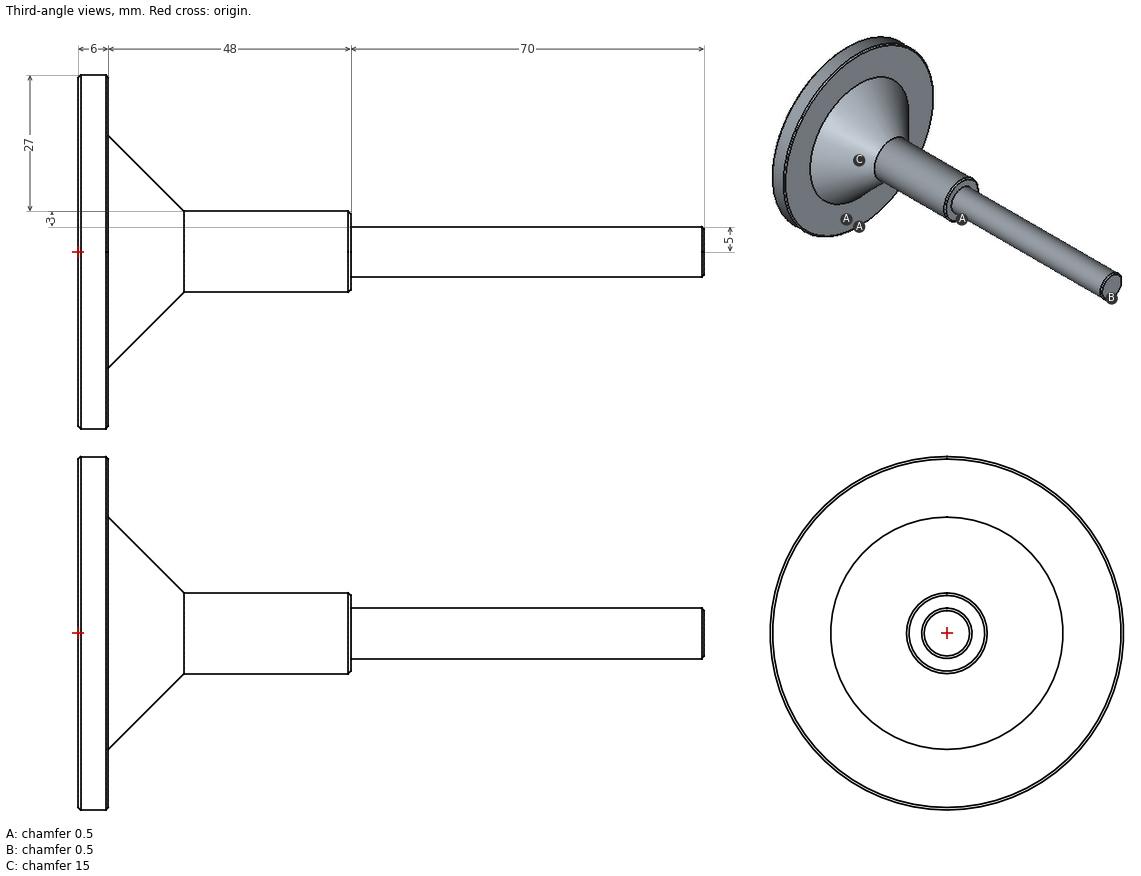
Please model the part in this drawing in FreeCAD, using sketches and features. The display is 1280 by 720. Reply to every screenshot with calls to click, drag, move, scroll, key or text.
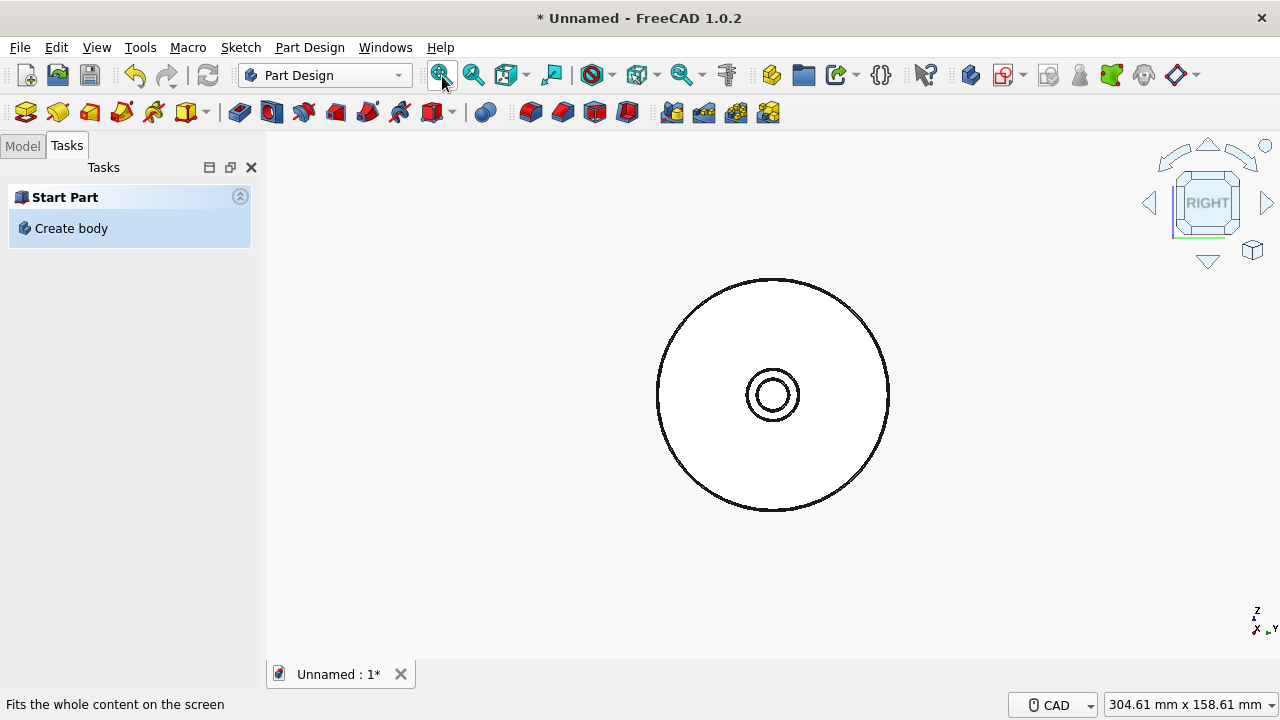
key(5)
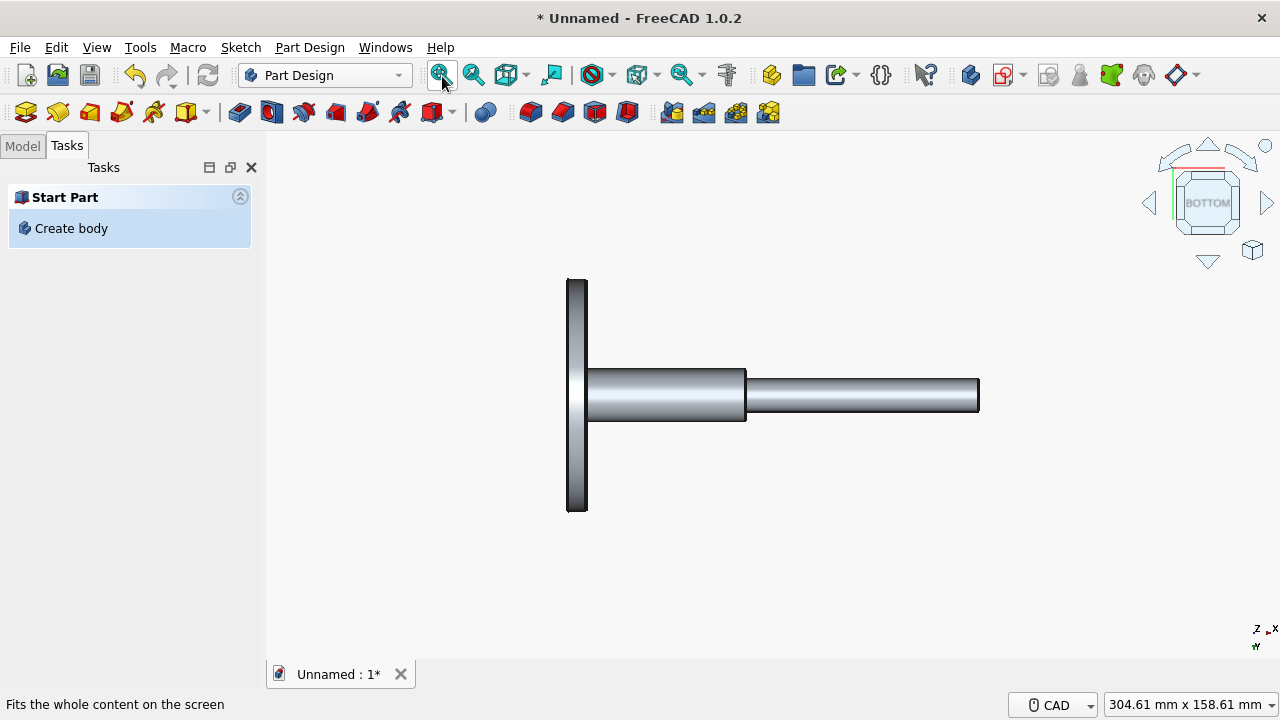
click(442, 76)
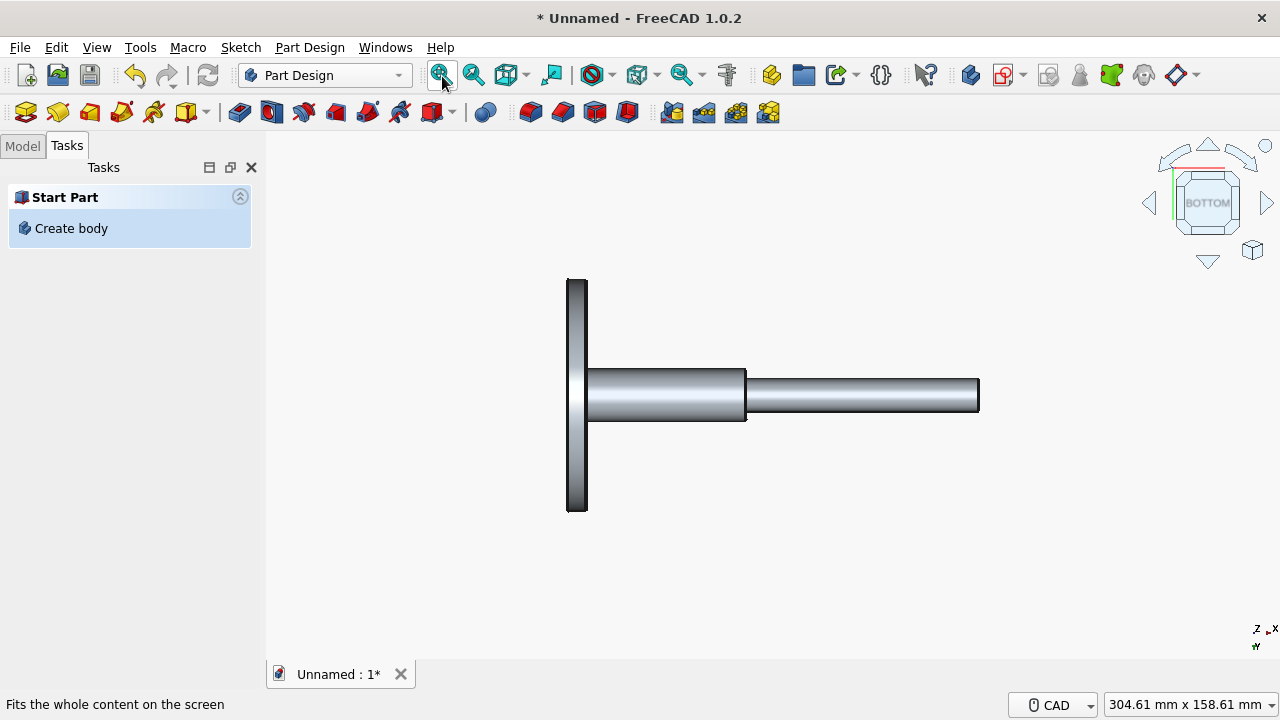
key(4)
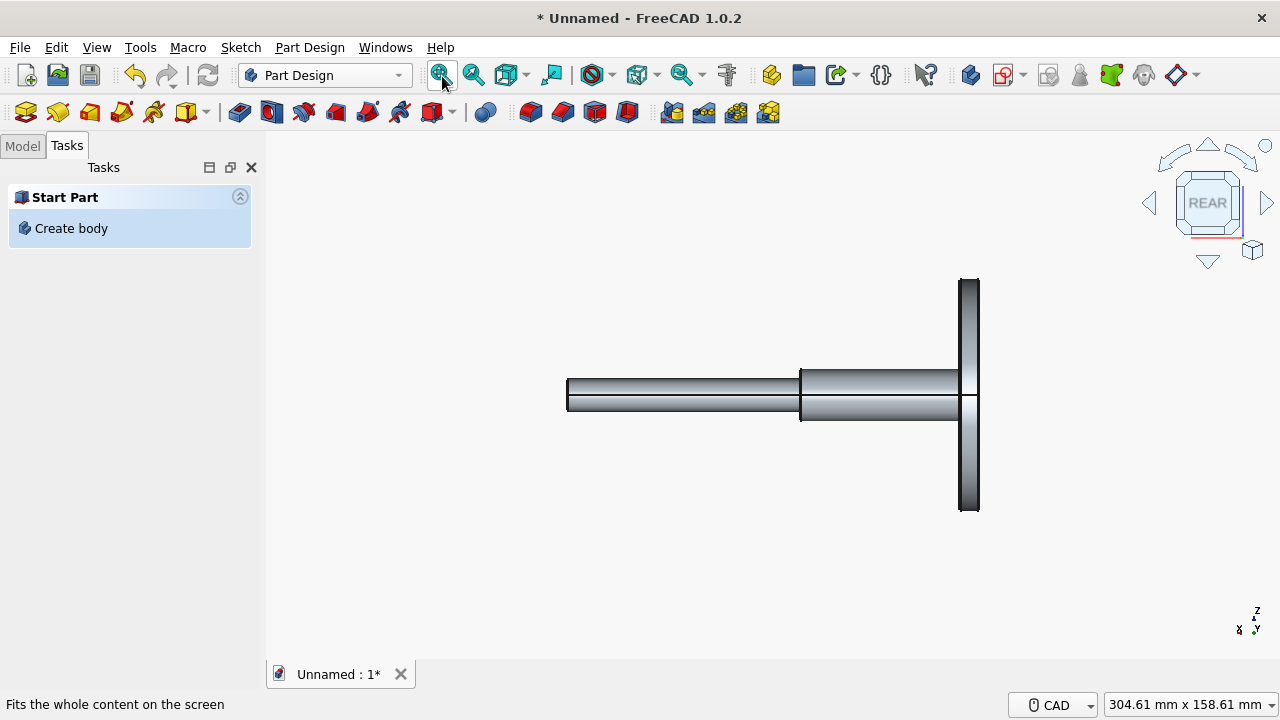
click(442, 76)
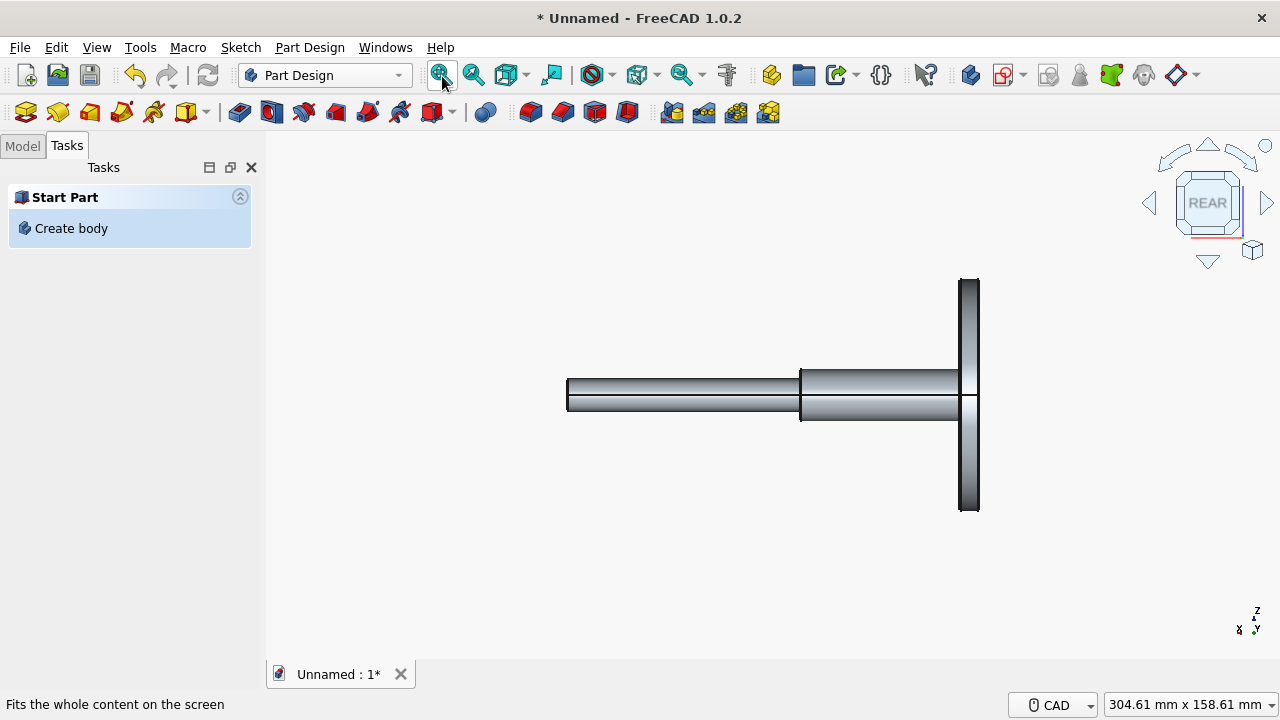
key(6)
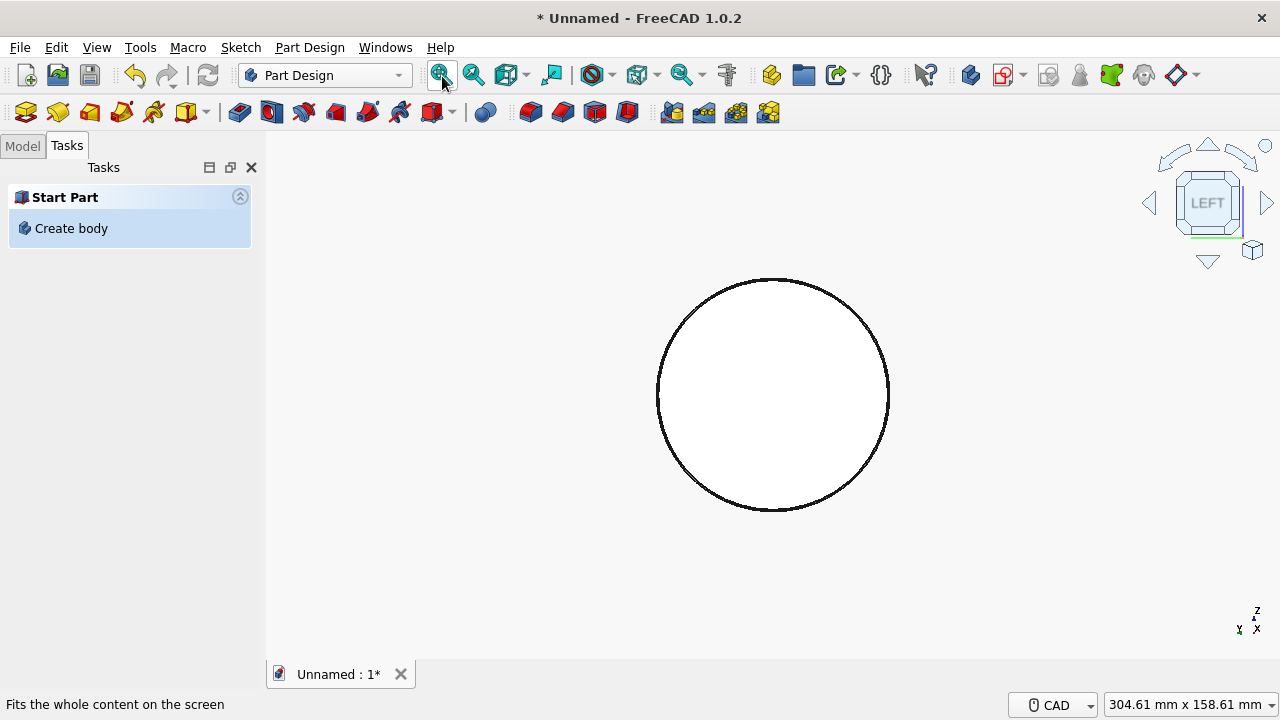
click(442, 76)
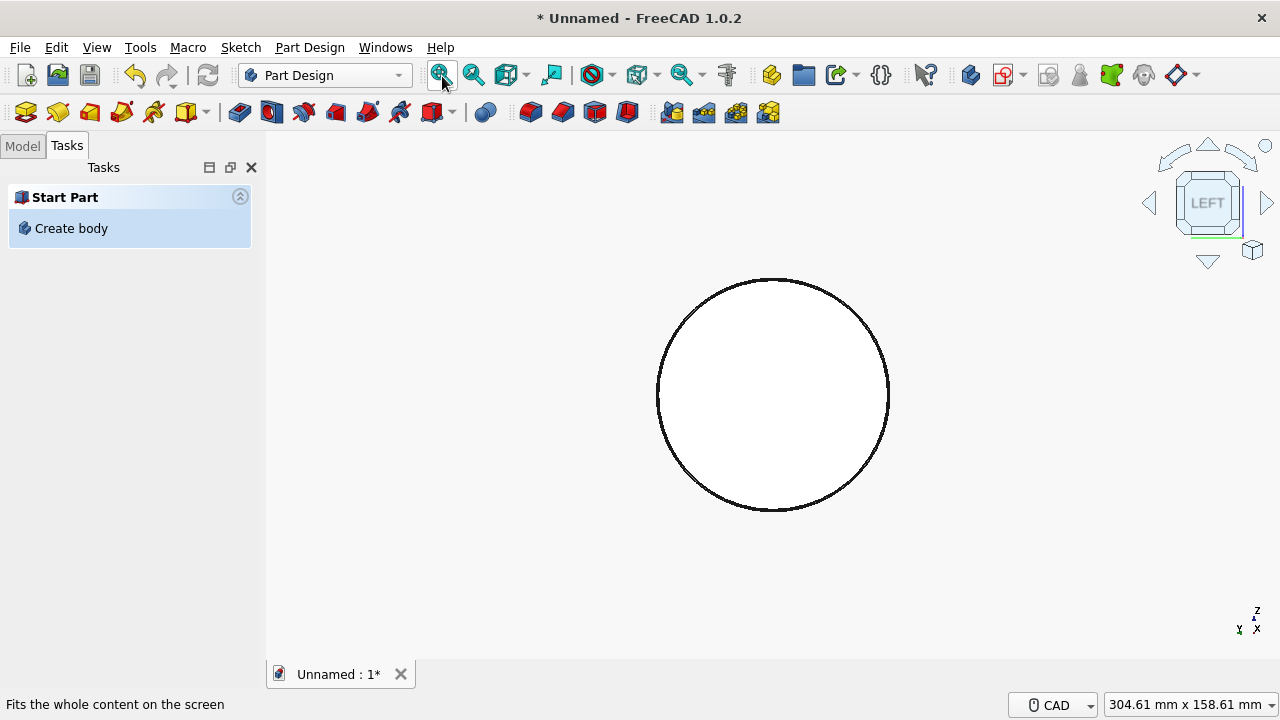
key(v)
key(3)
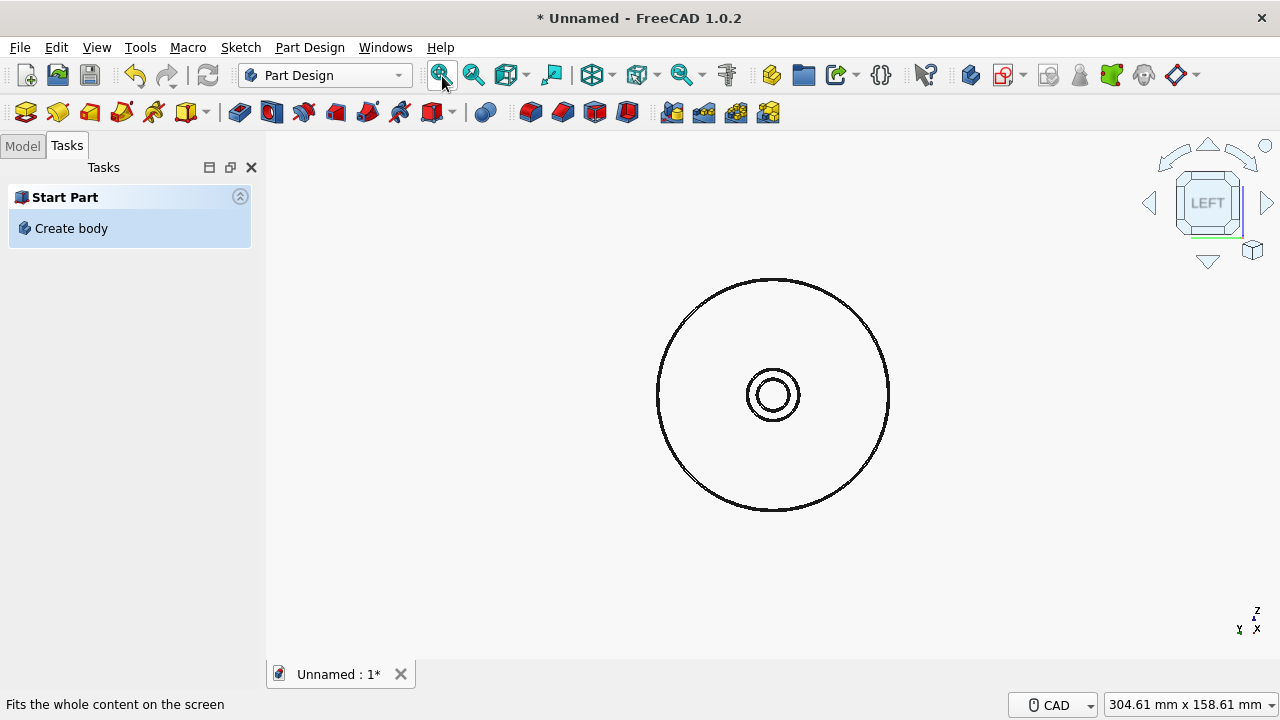
key(0)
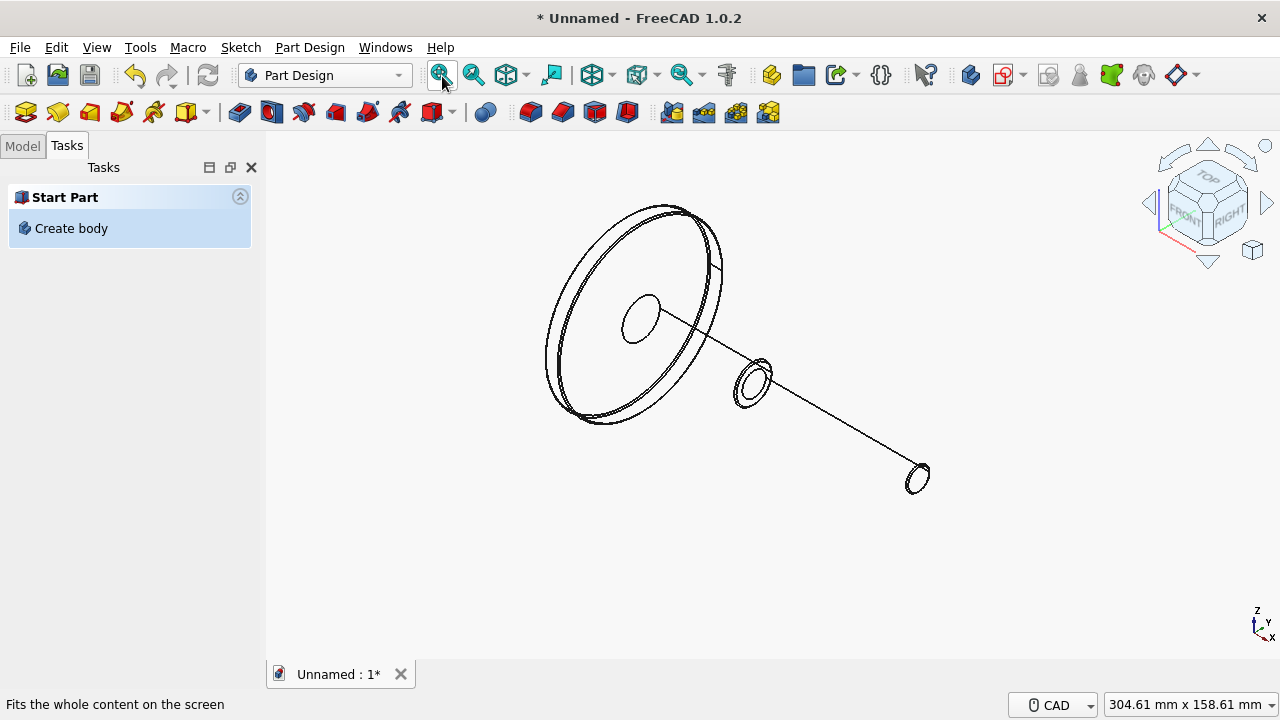
click(622, 329)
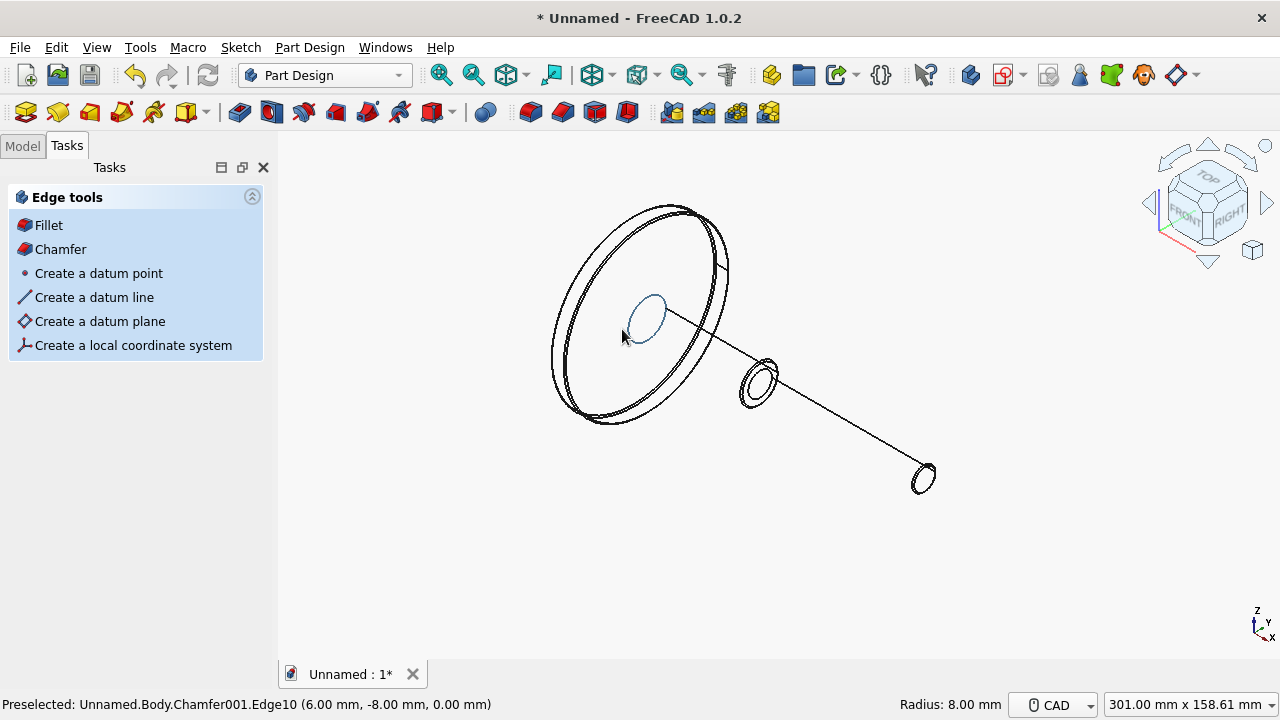
key(v)
key(1)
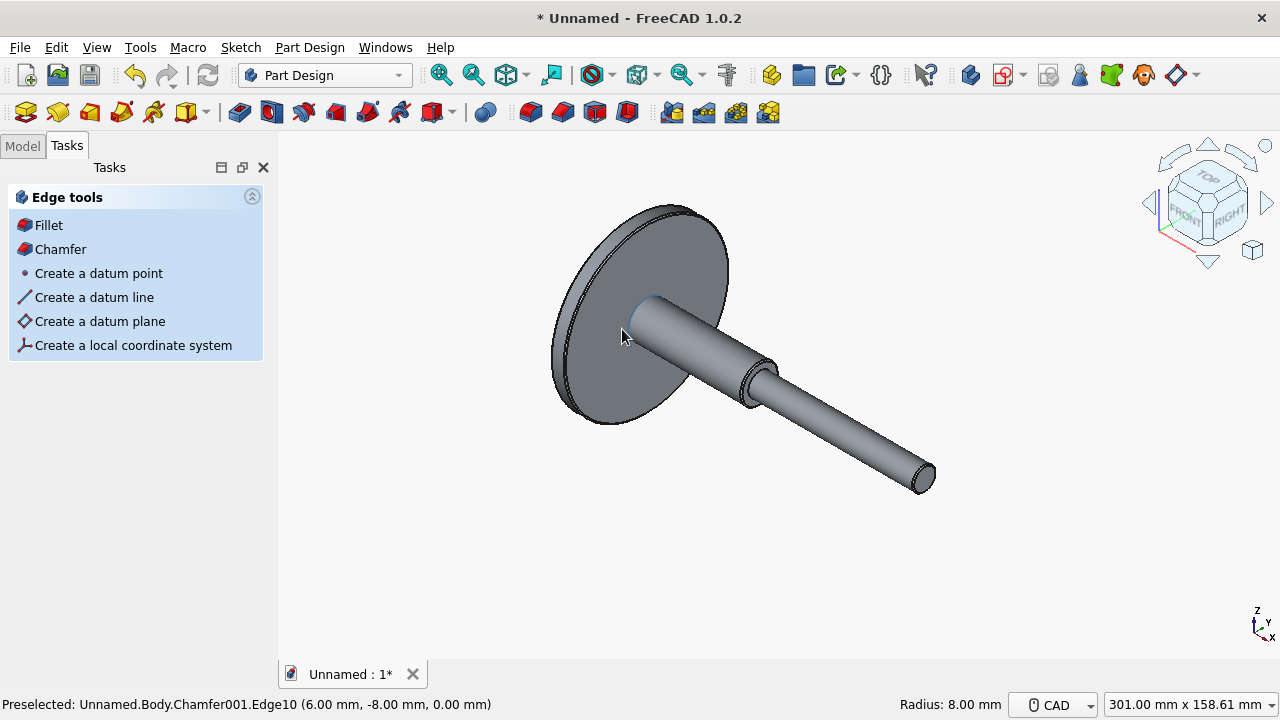
click(564, 112)